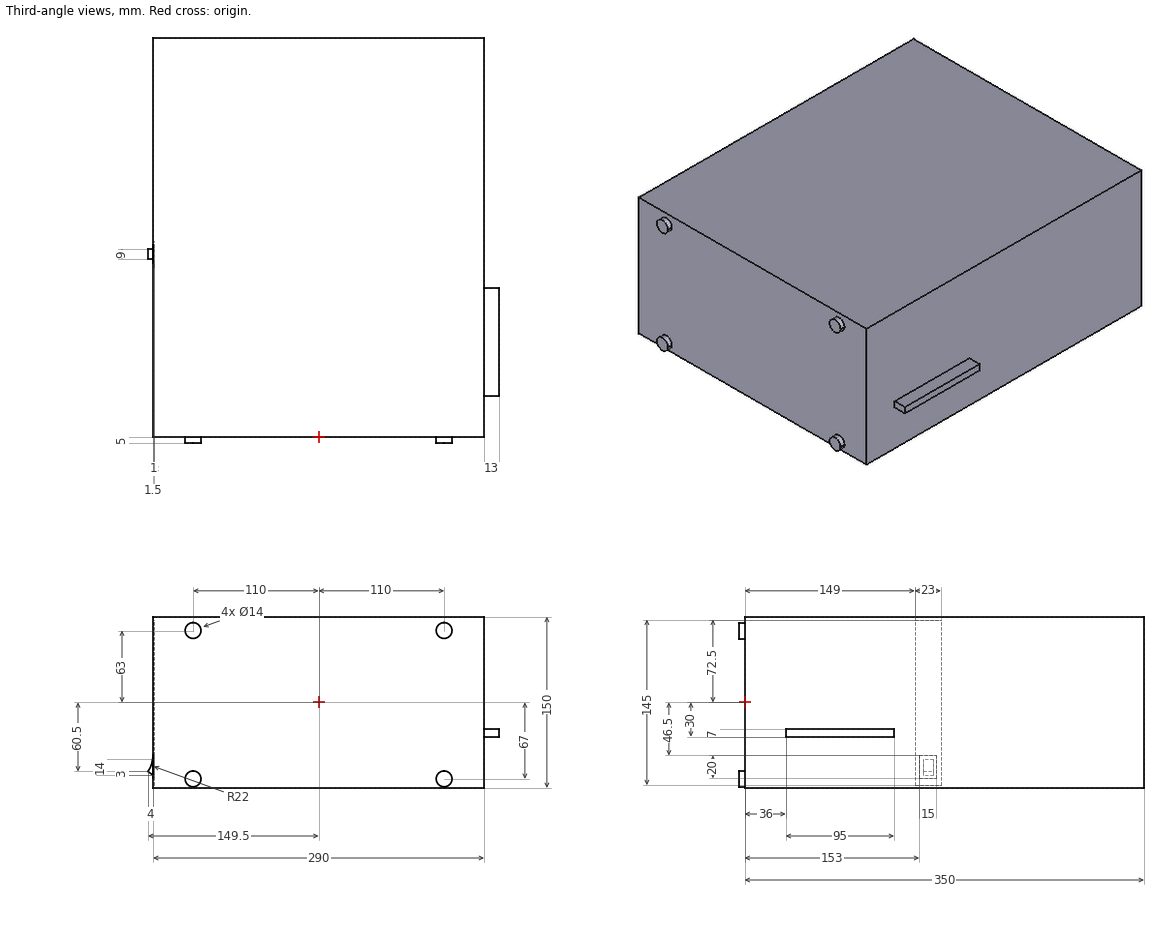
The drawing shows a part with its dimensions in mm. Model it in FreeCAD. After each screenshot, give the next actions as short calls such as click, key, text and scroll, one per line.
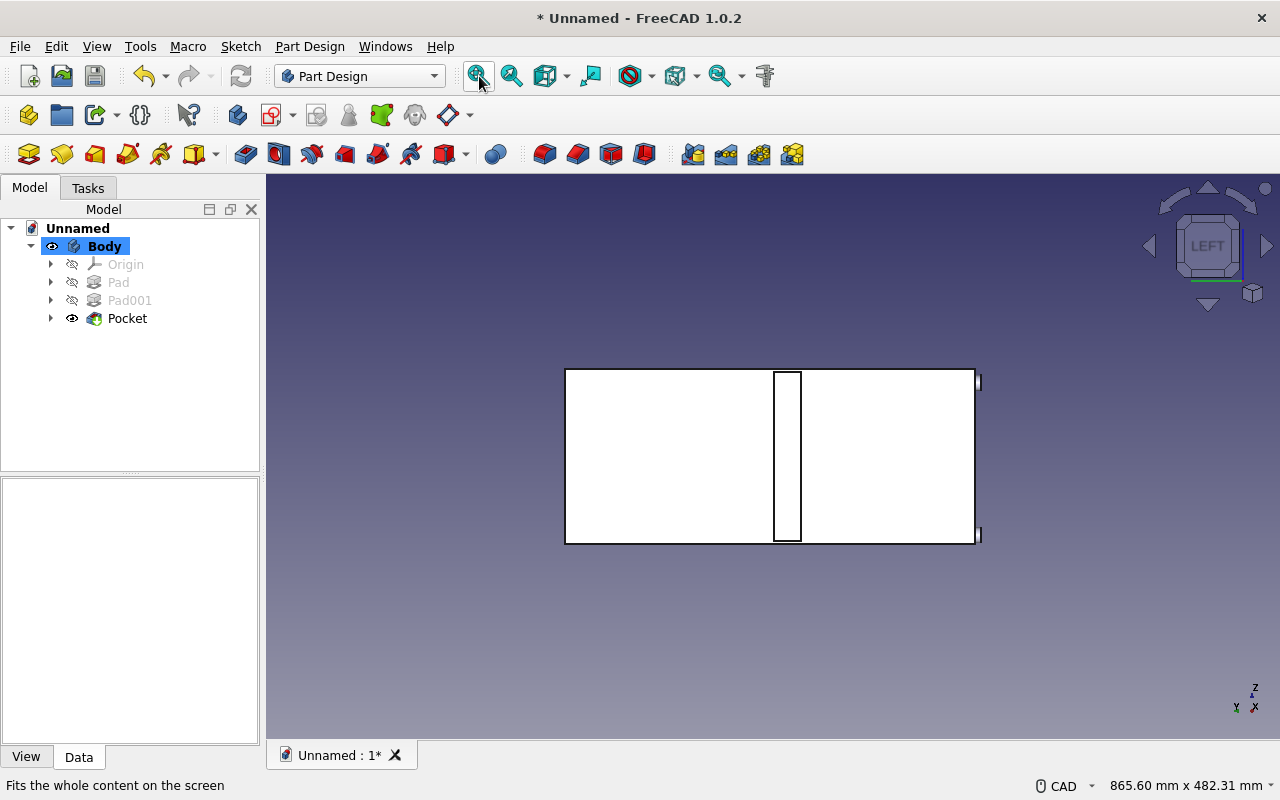
click(787, 504)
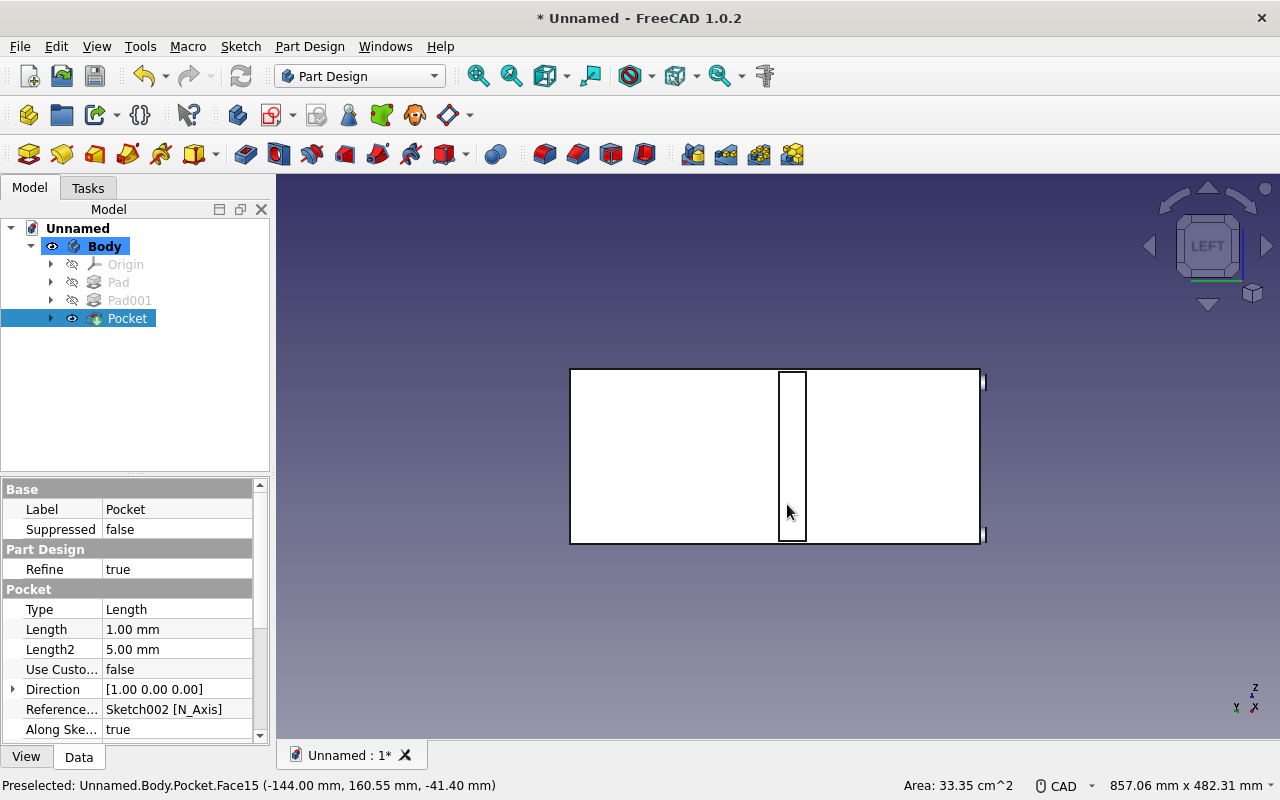
click(270, 116)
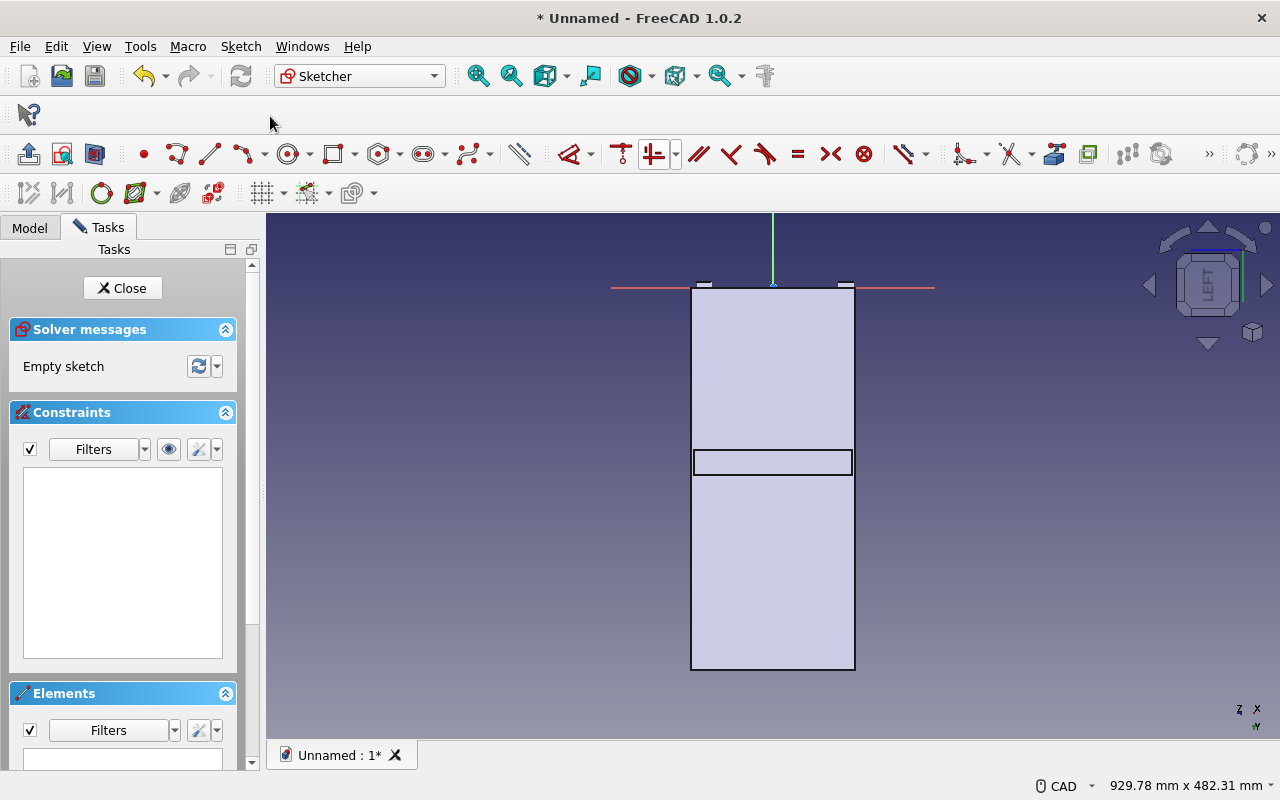
click(95, 154)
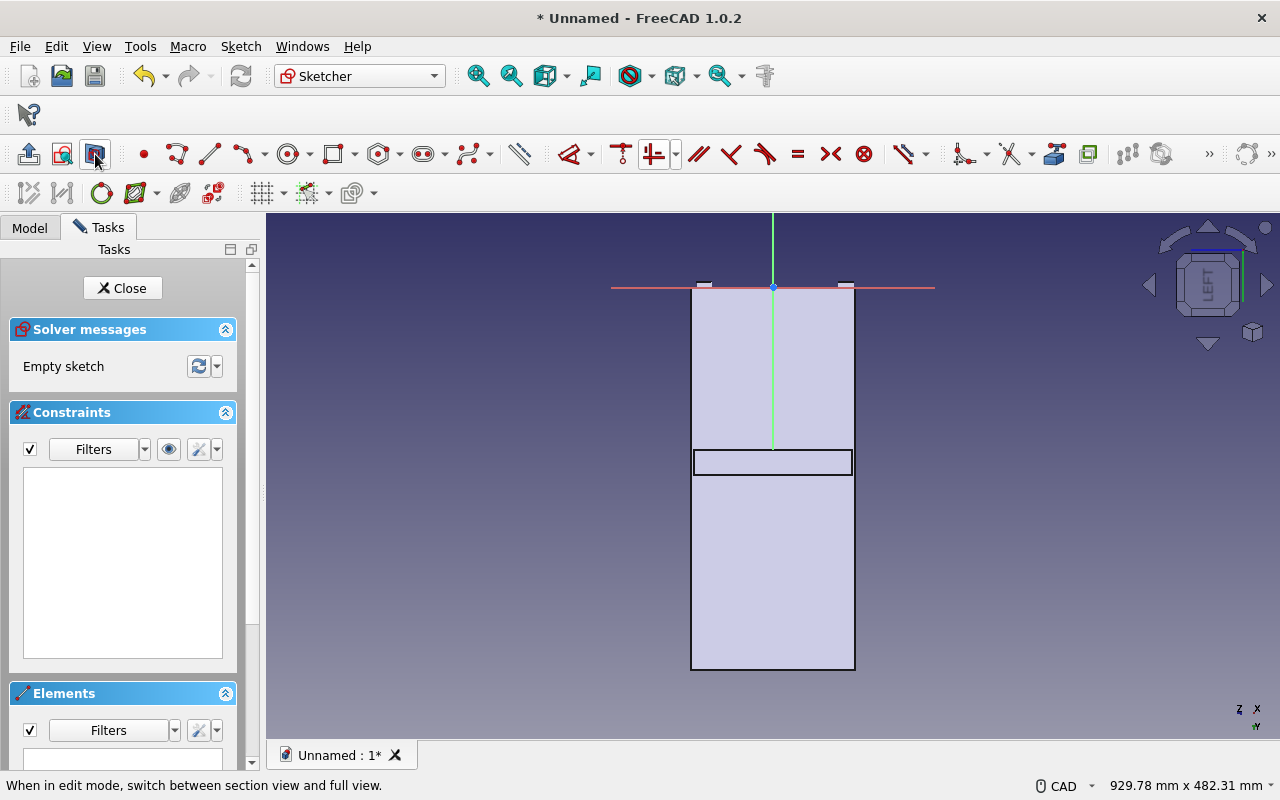
scroll(841, 462, up, 15)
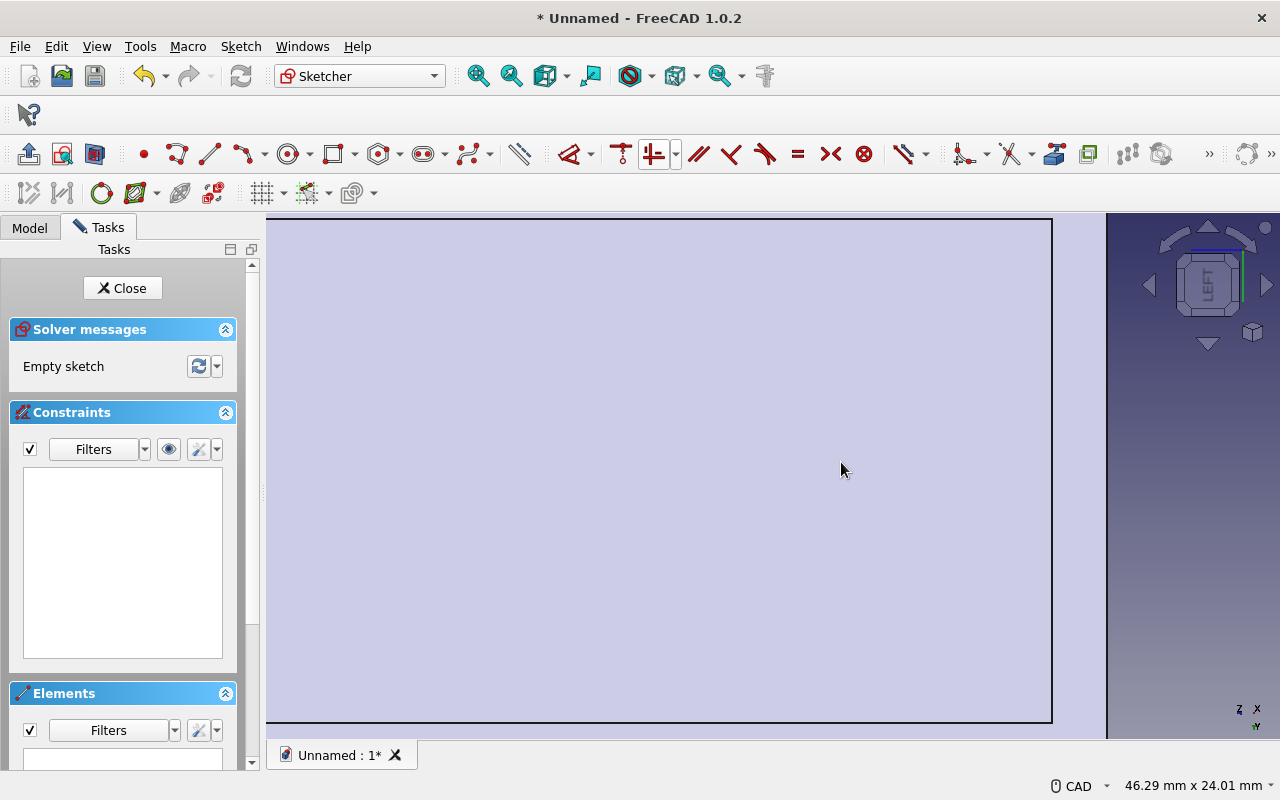
click(332, 154)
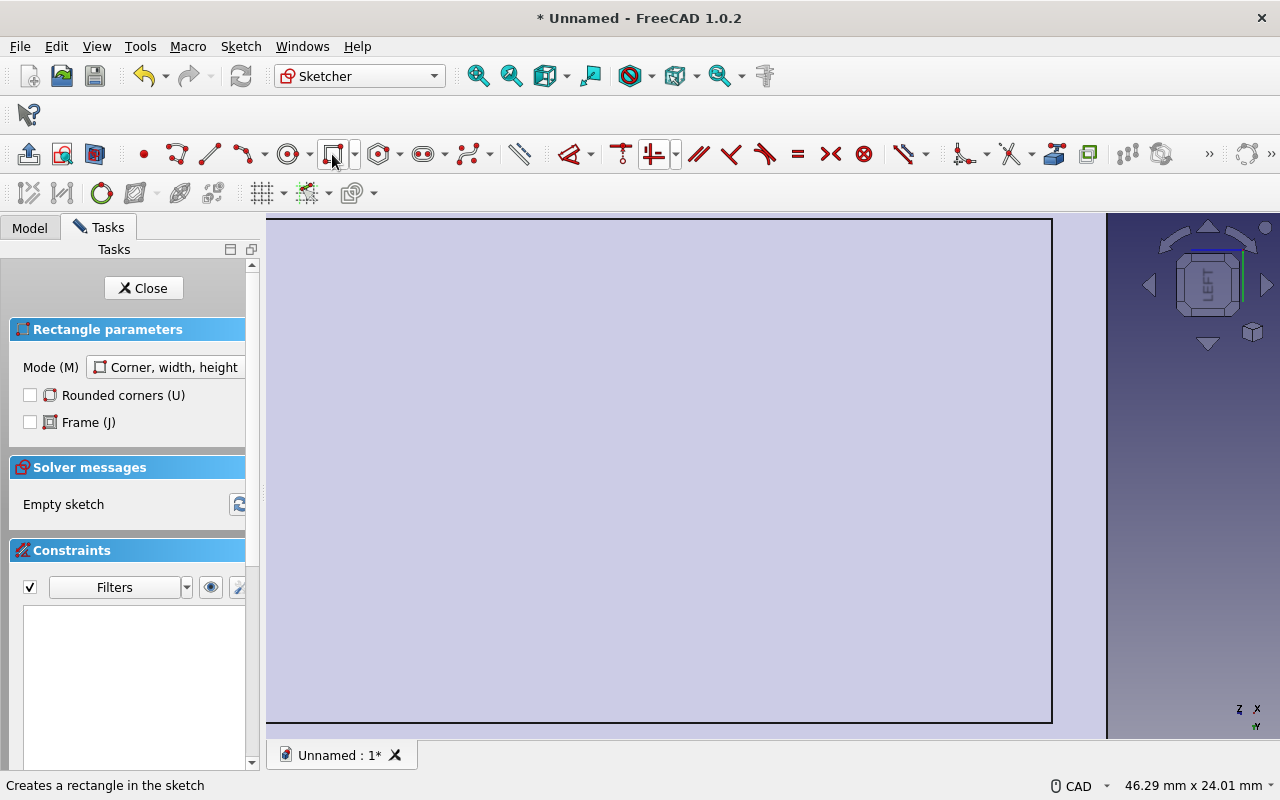
click(483, 307)
click(921, 636)
key(Escape)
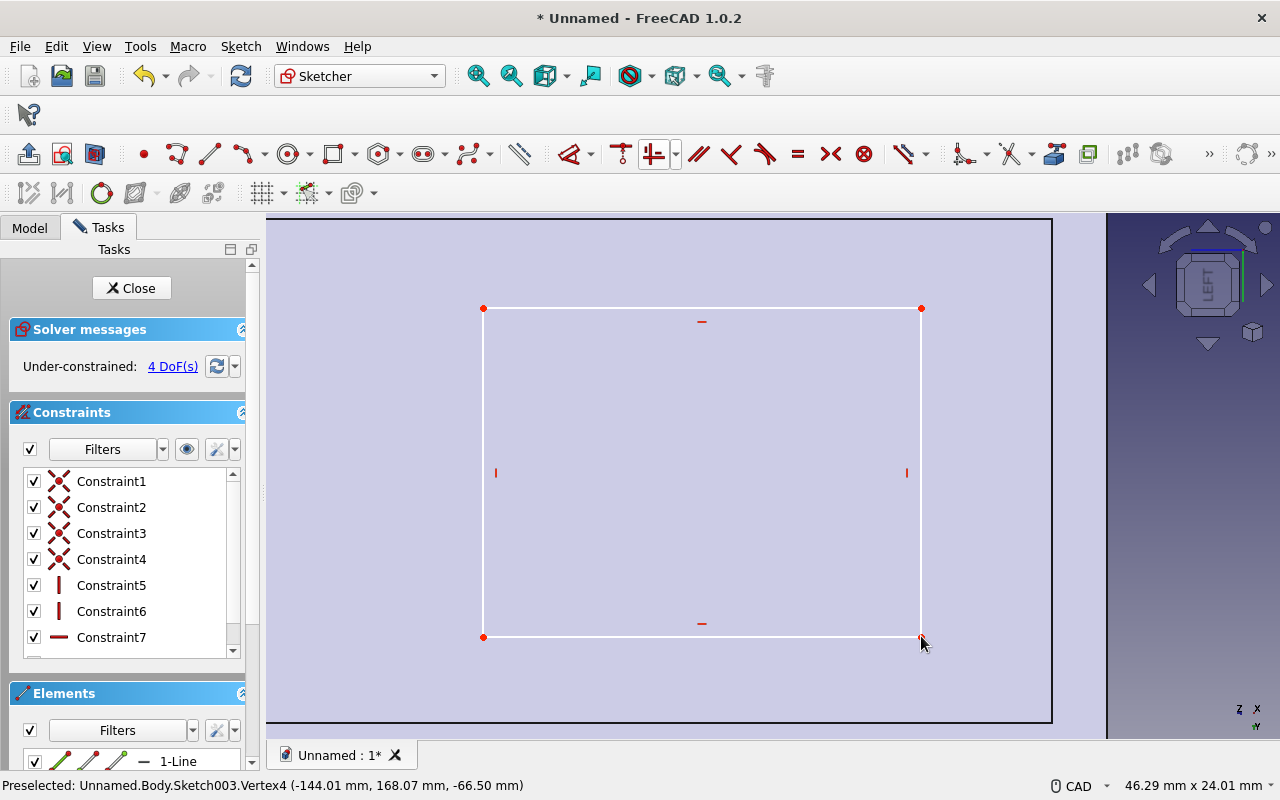
click(568, 154)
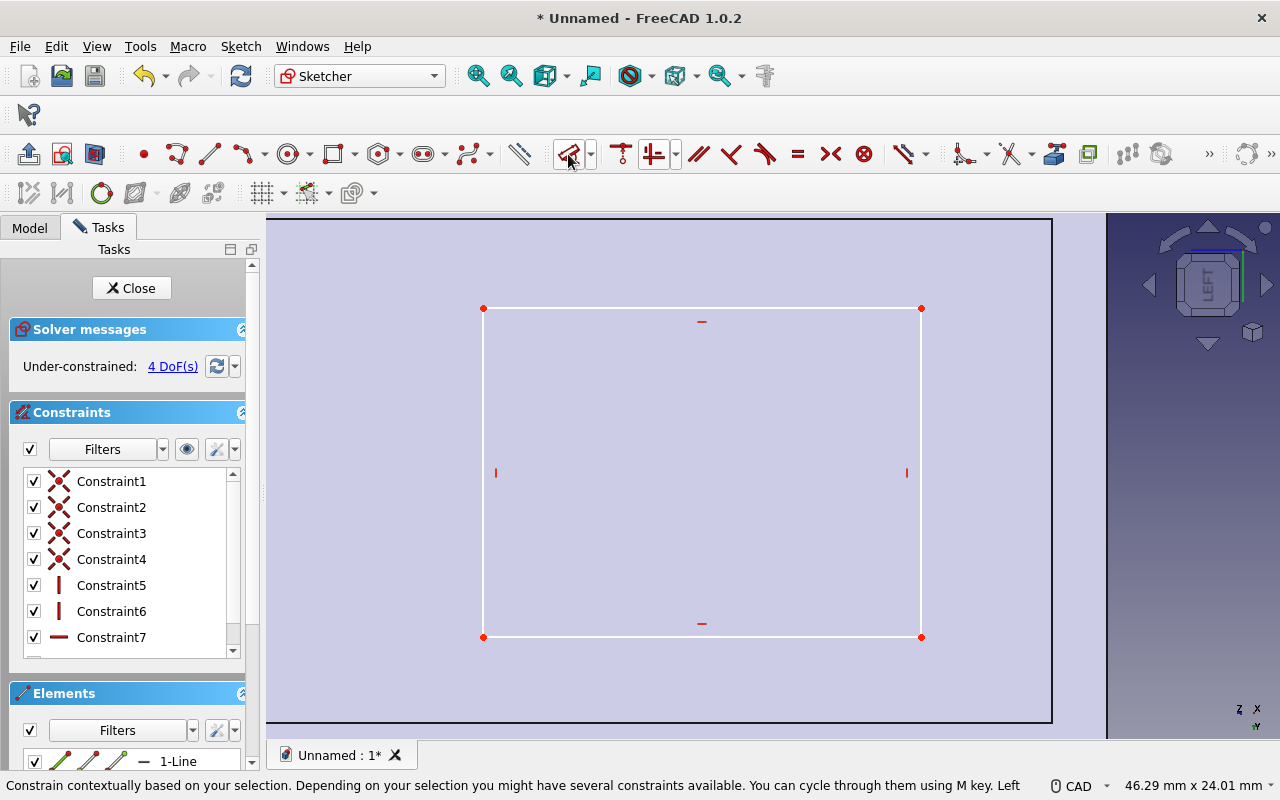
click(483, 407)
click(449, 472)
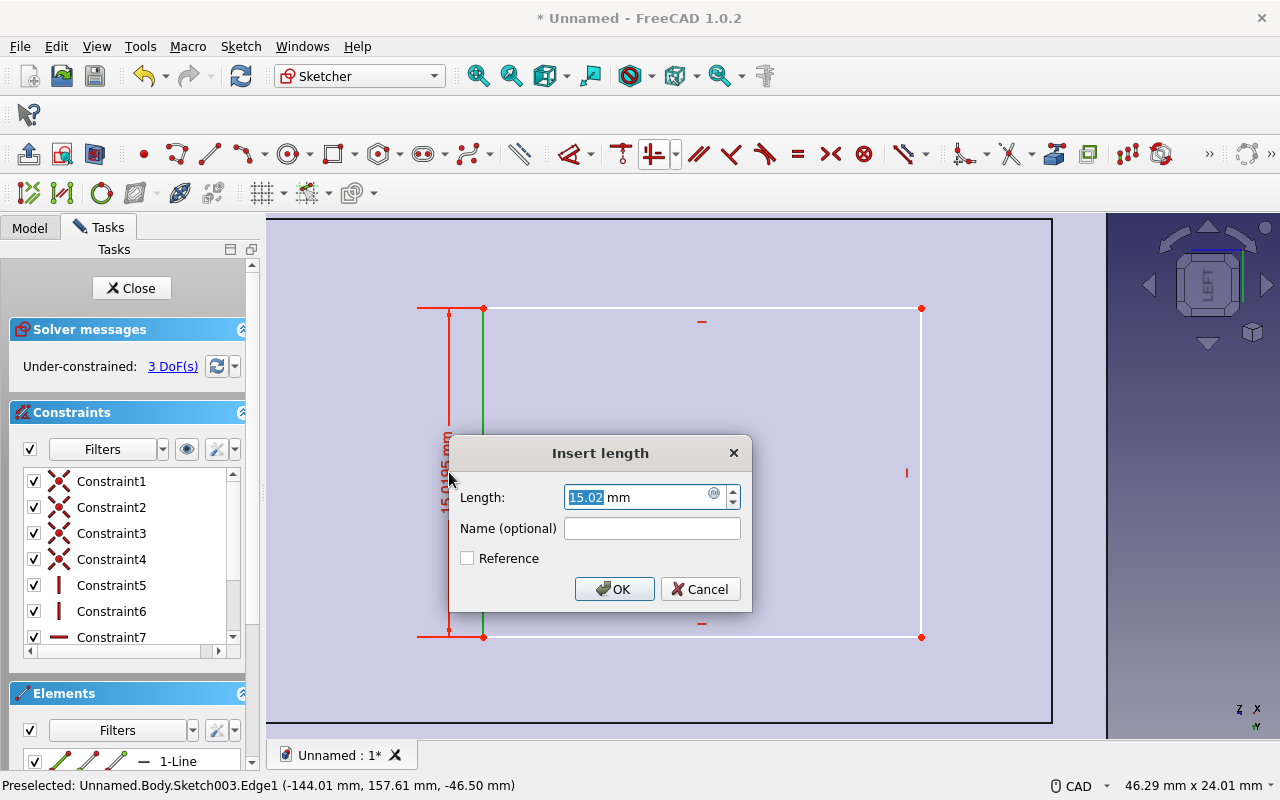
text(15)
key(Return)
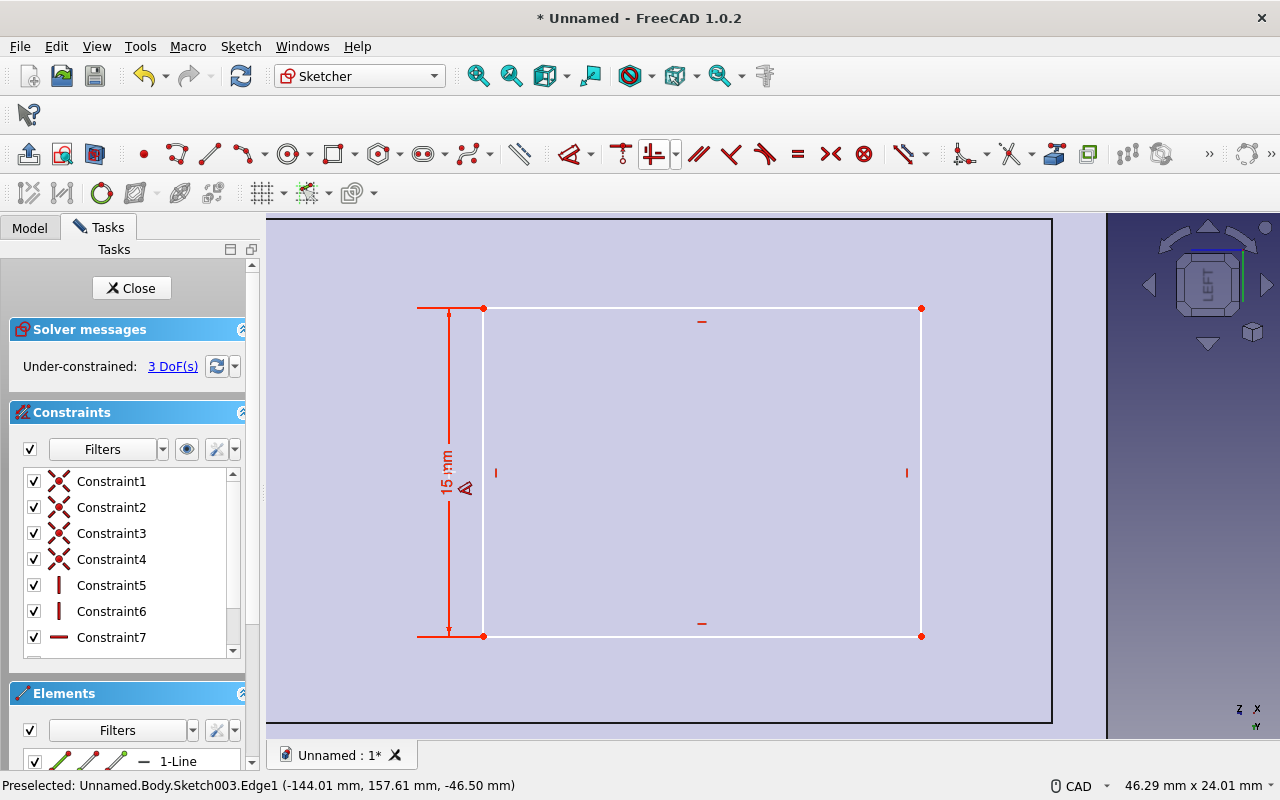
click(614, 637)
click(702, 671)